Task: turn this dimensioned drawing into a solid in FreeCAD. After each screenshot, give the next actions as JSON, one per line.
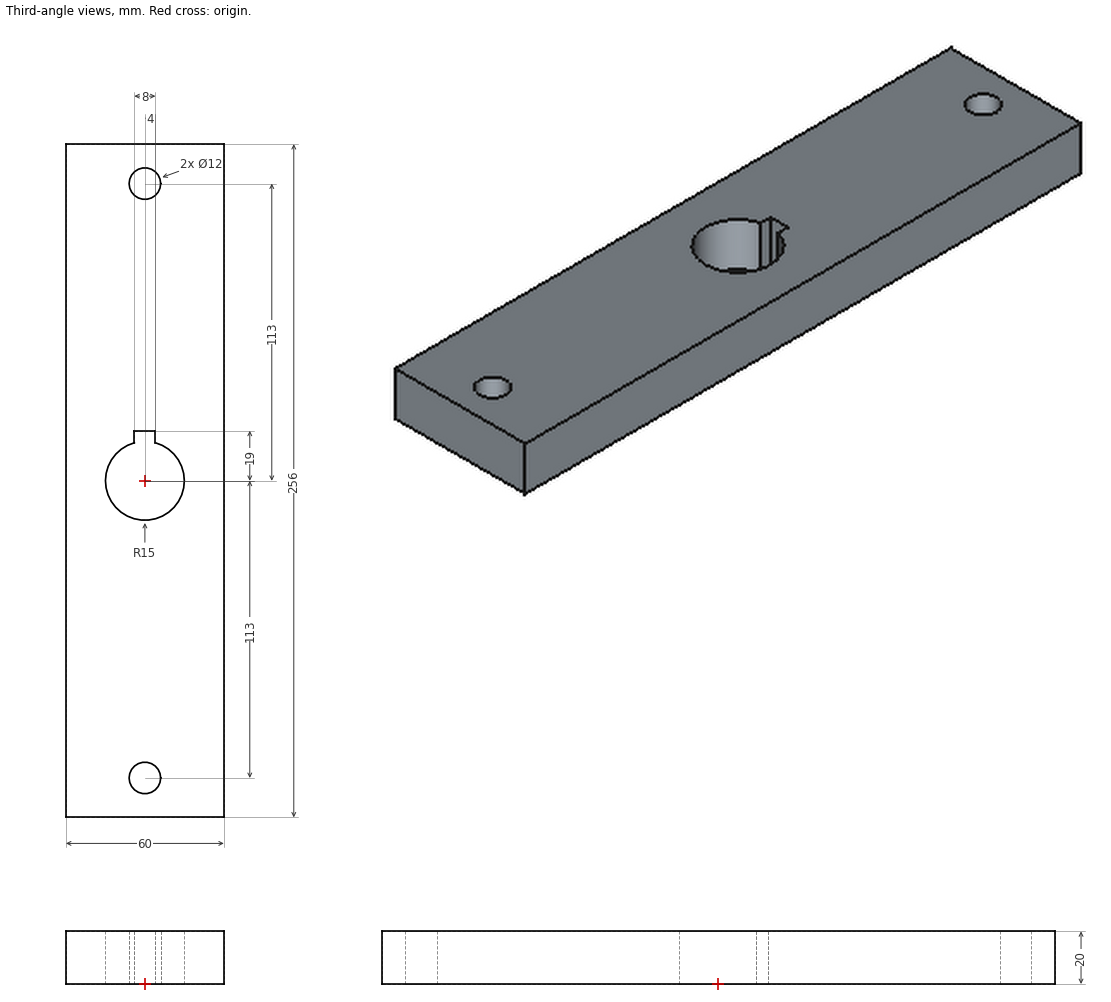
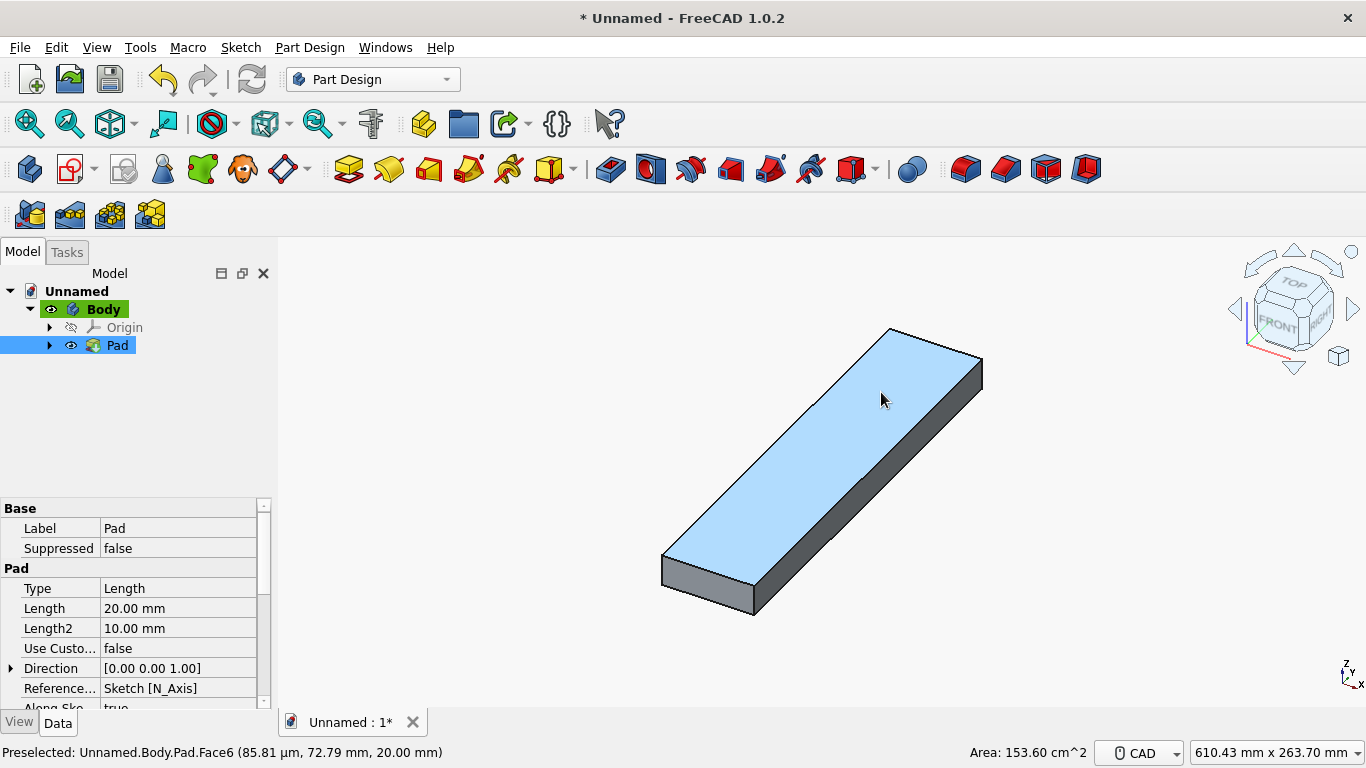
{"action": "left_click", "coordinate": [70, 170]}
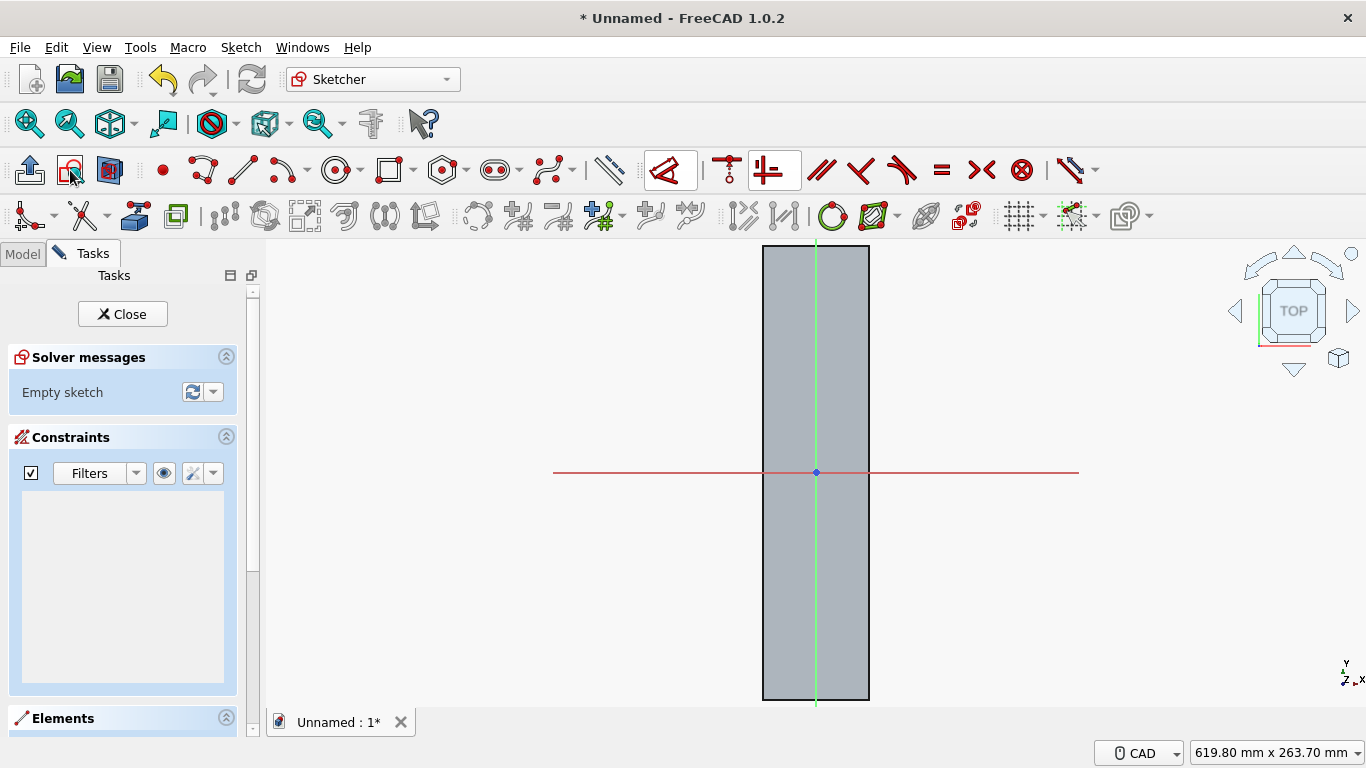
{"action": "scroll", "coordinate": [608, 473], "scroll_direction": "down", "scroll_amount": 2}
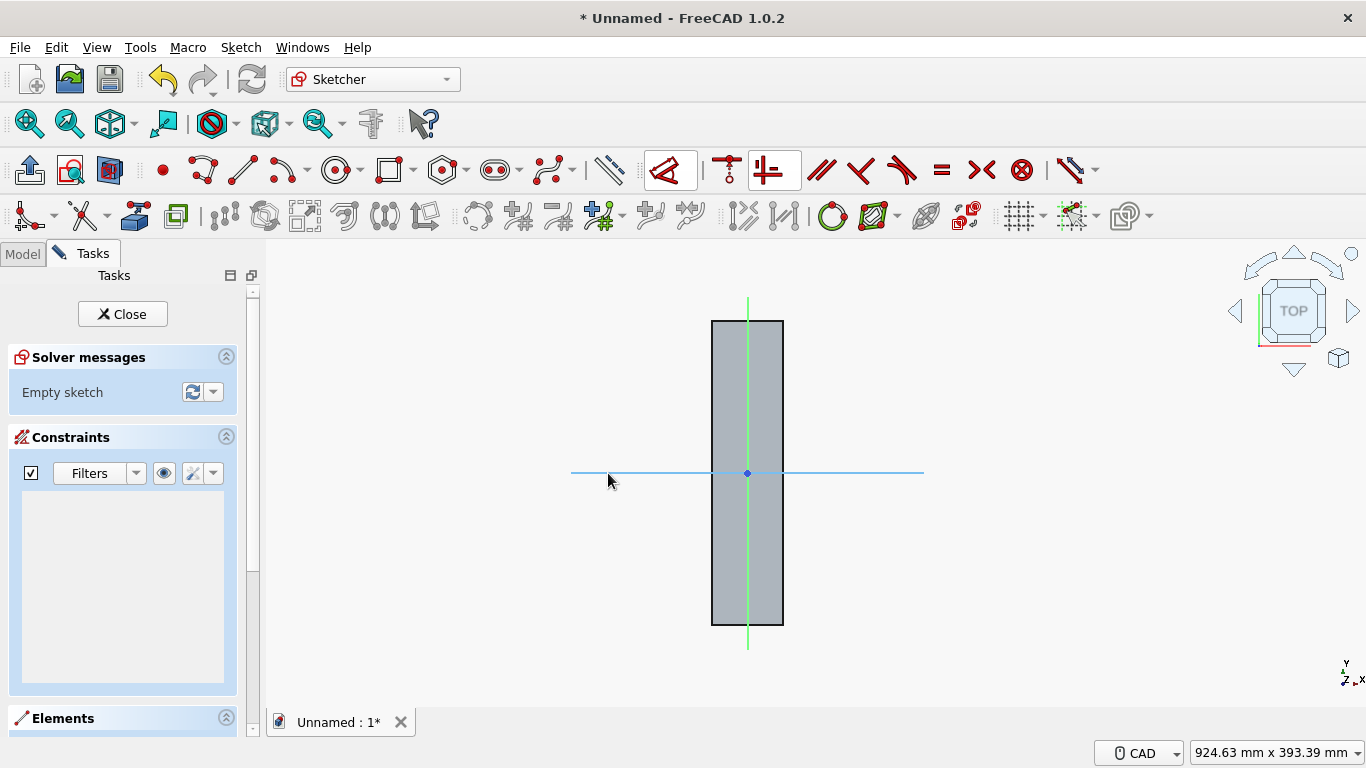
{"action": "left_click", "coordinate": [336, 170]}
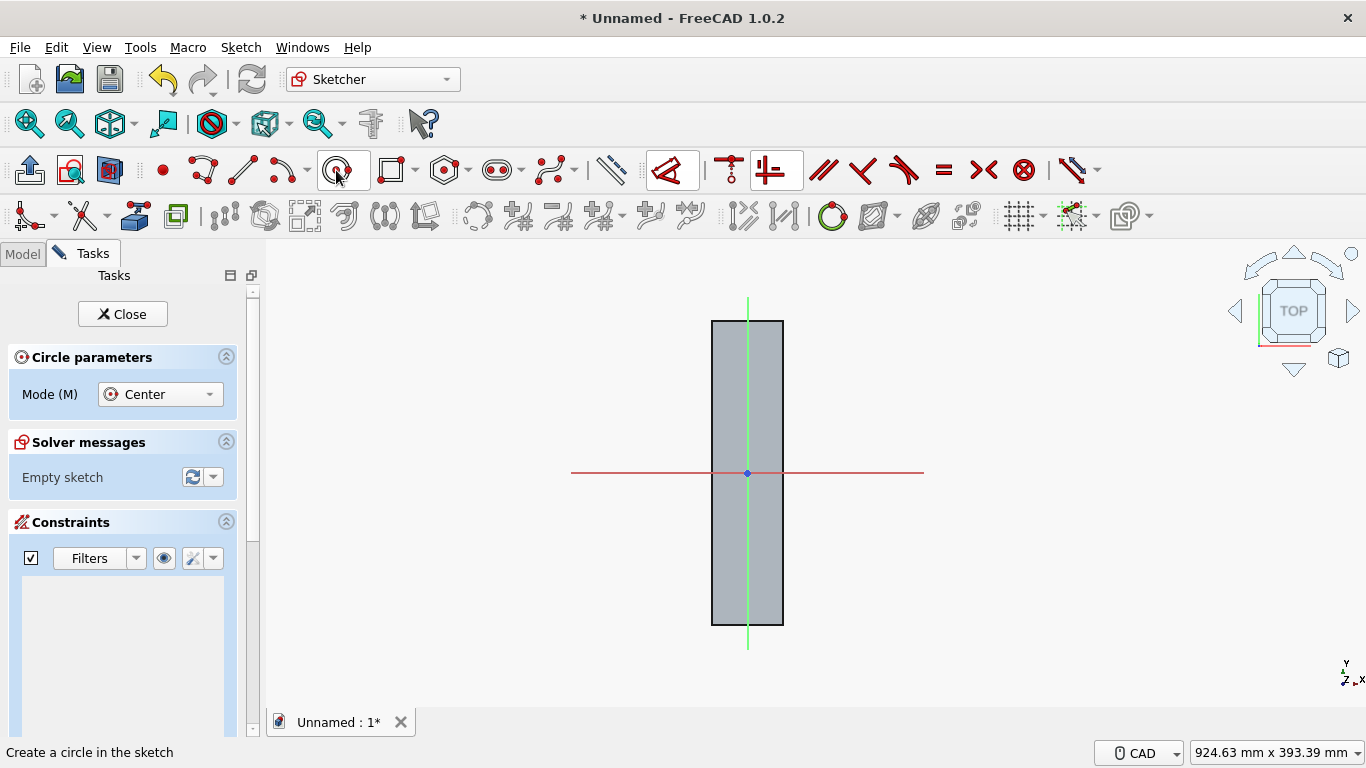
{"action": "scroll", "coordinate": [748, 339], "scroll_direction": "up", "scroll_amount": 6}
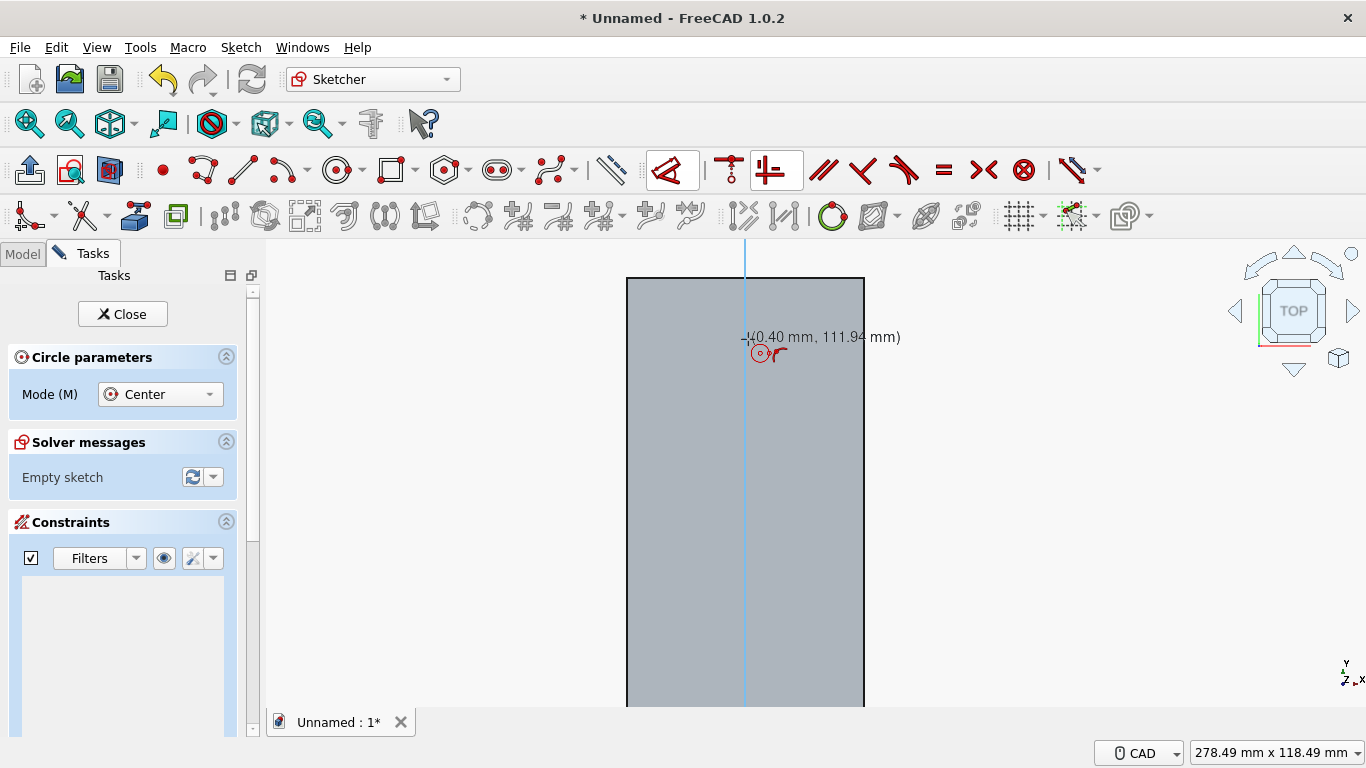
{"action": "left_click", "coordinate": [745, 338]}
{"action": "left_click", "coordinate": [762, 321]}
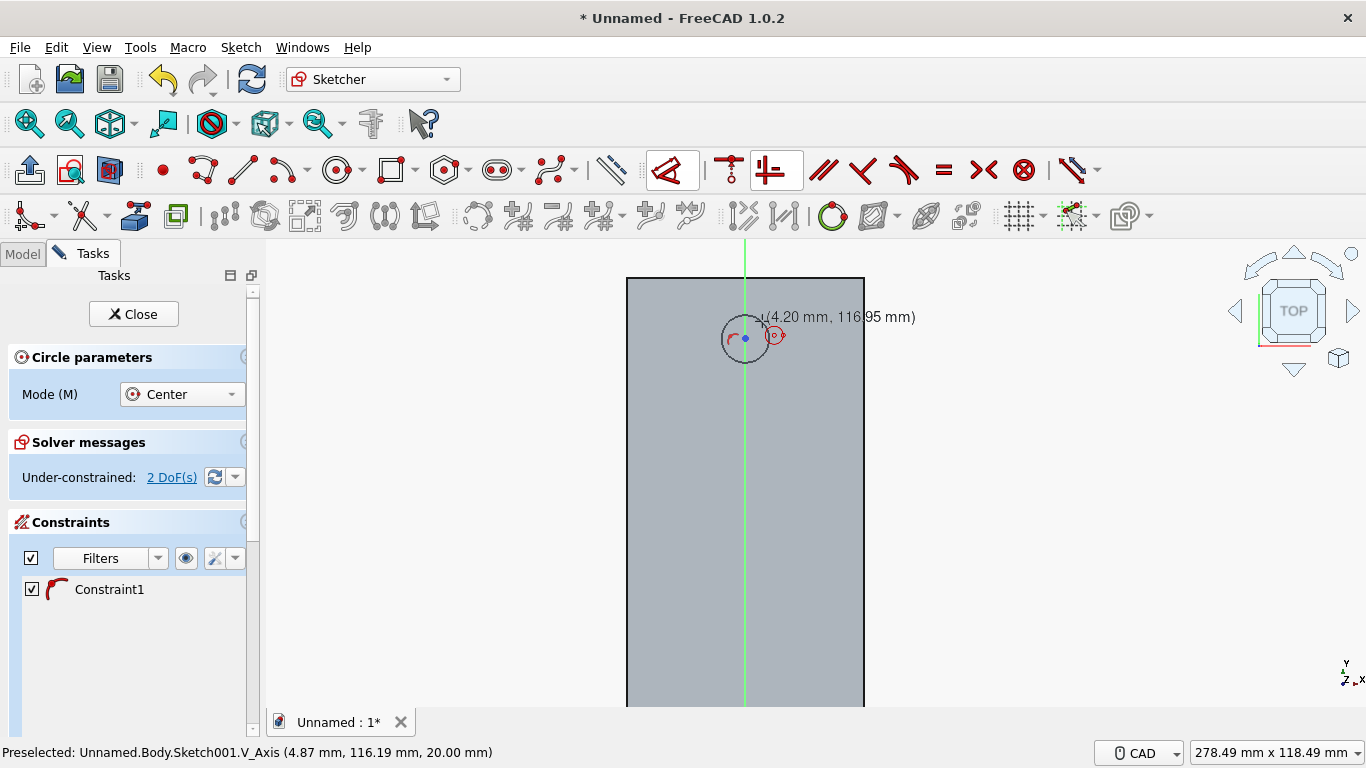
{"action": "scroll", "coordinate": [748, 339], "scroll_direction": "down", "scroll_amount": 6}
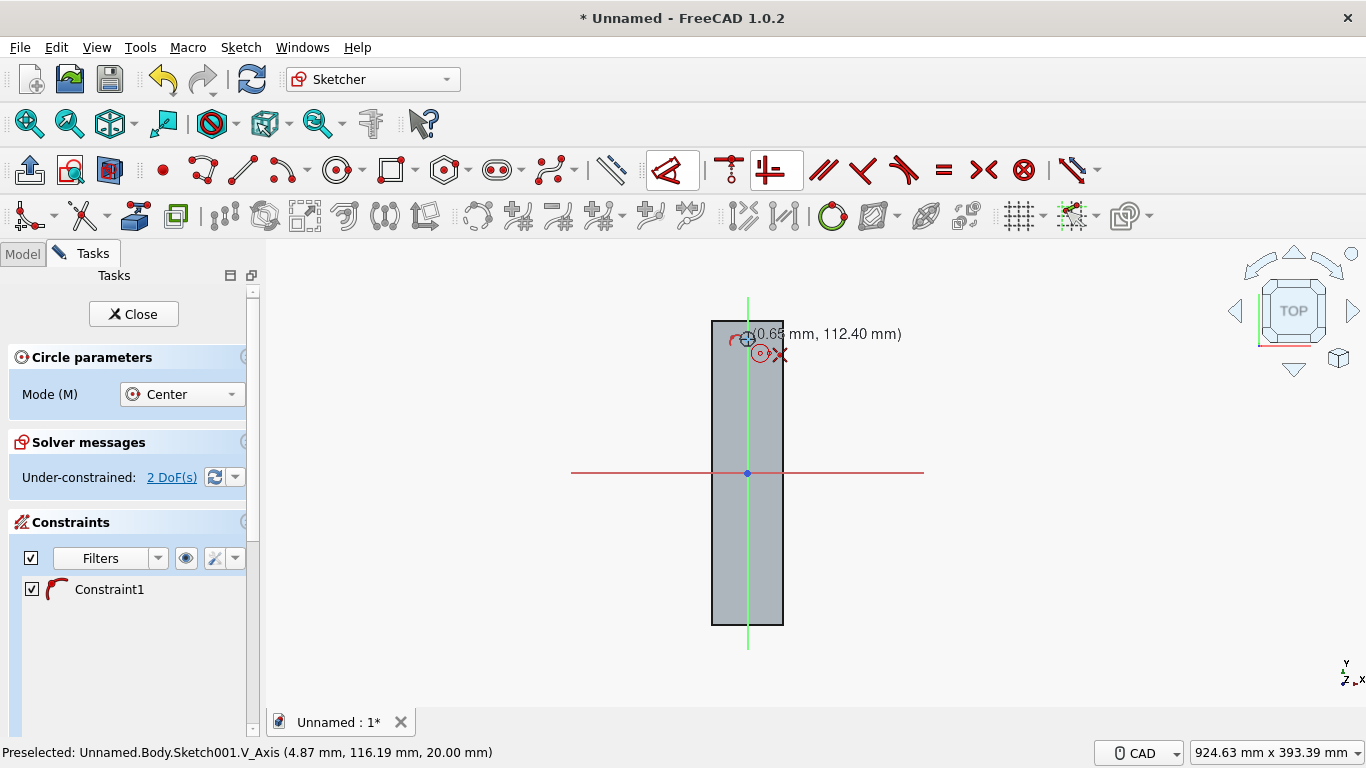
{"action": "scroll", "coordinate": [748, 608], "scroll_direction": "up", "scroll_amount": 6}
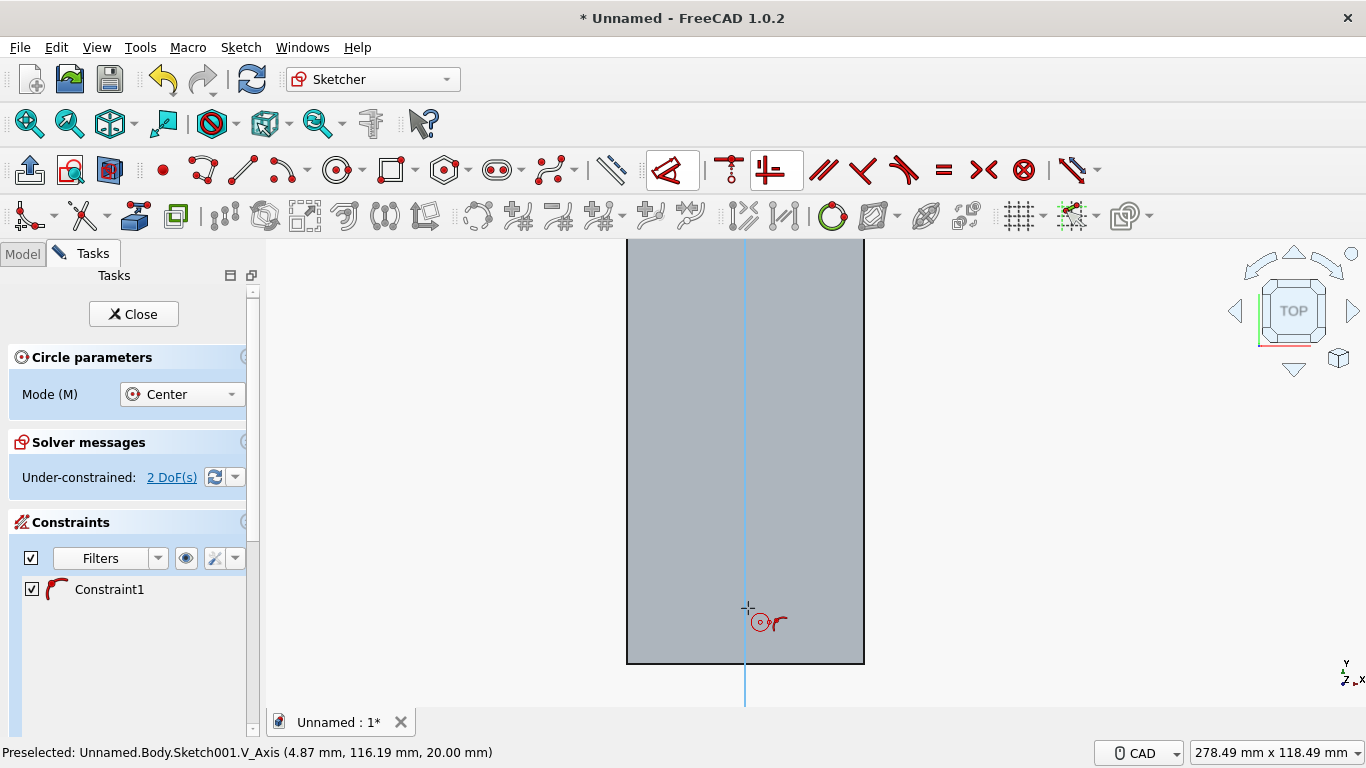
{"action": "left_click", "coordinate": [745, 605]}
{"action": "left_click", "coordinate": [762, 588]}
{"action": "key", "text": "Escape"}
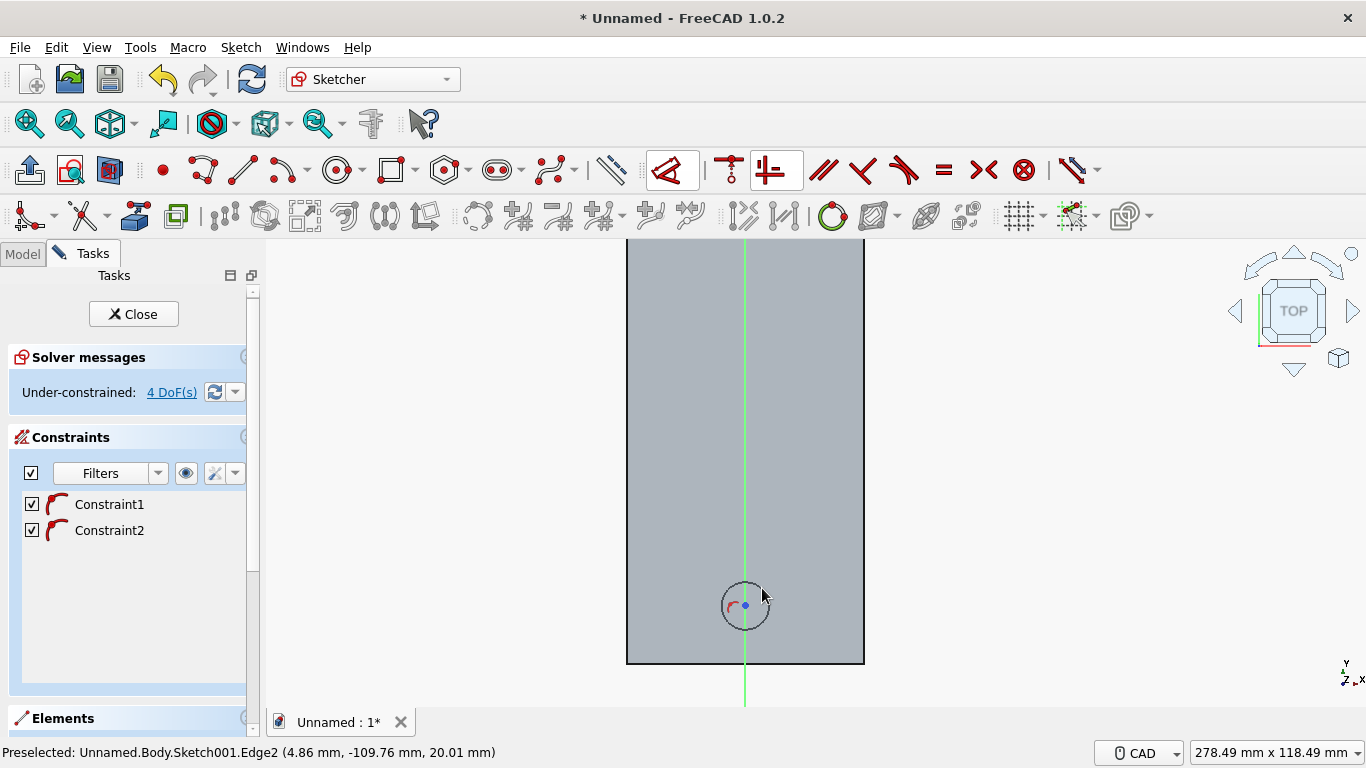
{"action": "scroll", "coordinate": [748, 609], "scroll_direction": "down", "scroll_amount": 6}